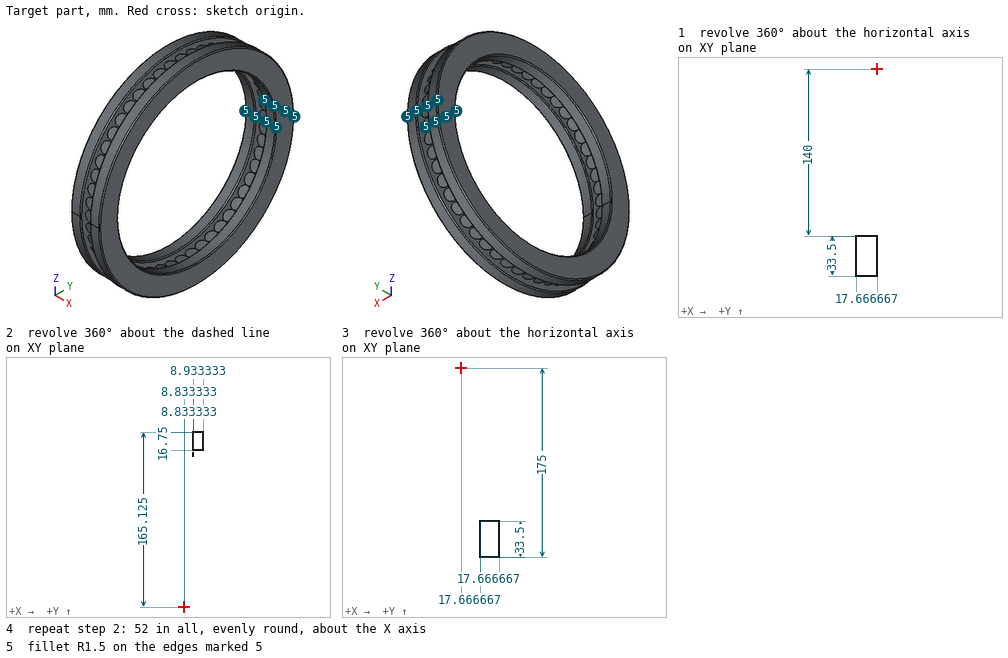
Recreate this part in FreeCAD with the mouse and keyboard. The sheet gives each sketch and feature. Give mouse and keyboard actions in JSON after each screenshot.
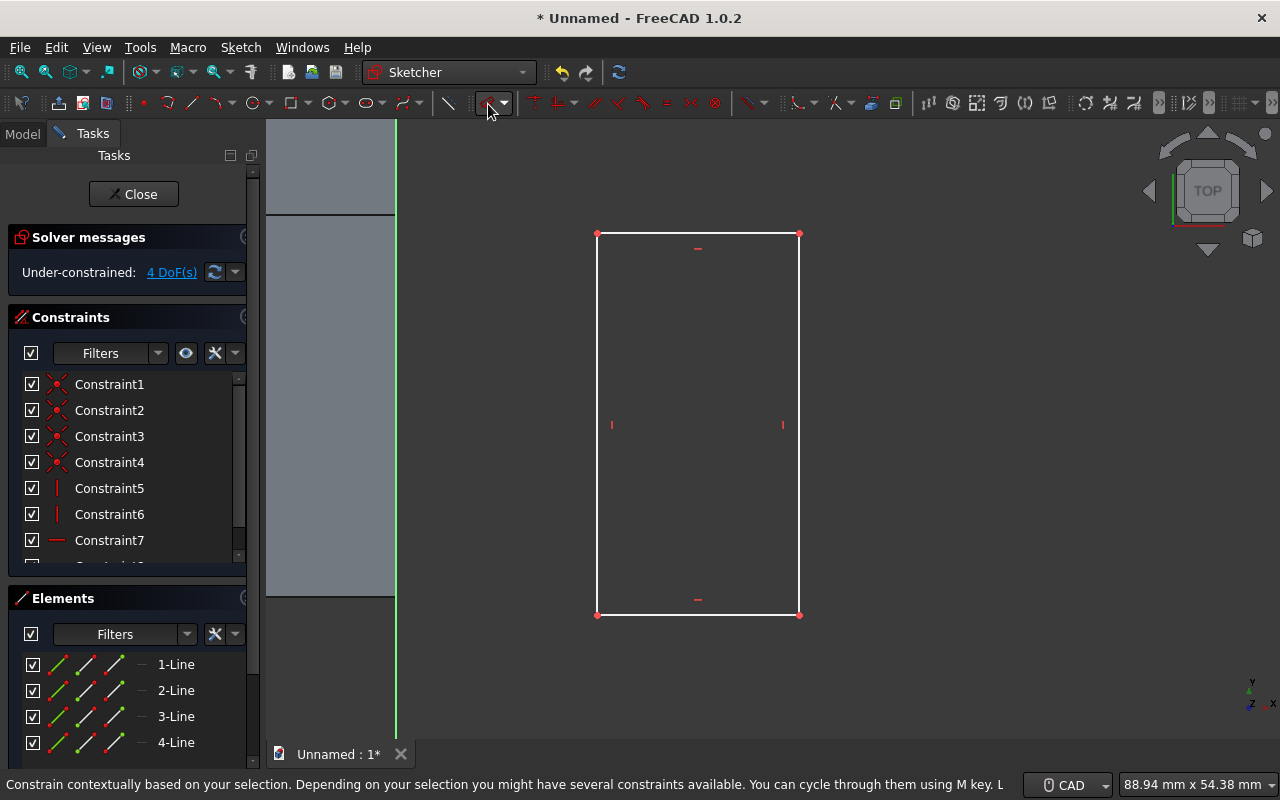
{"action": "left_click", "coordinate": [597, 348]}
{"action": "left_click", "coordinate": [563, 424]}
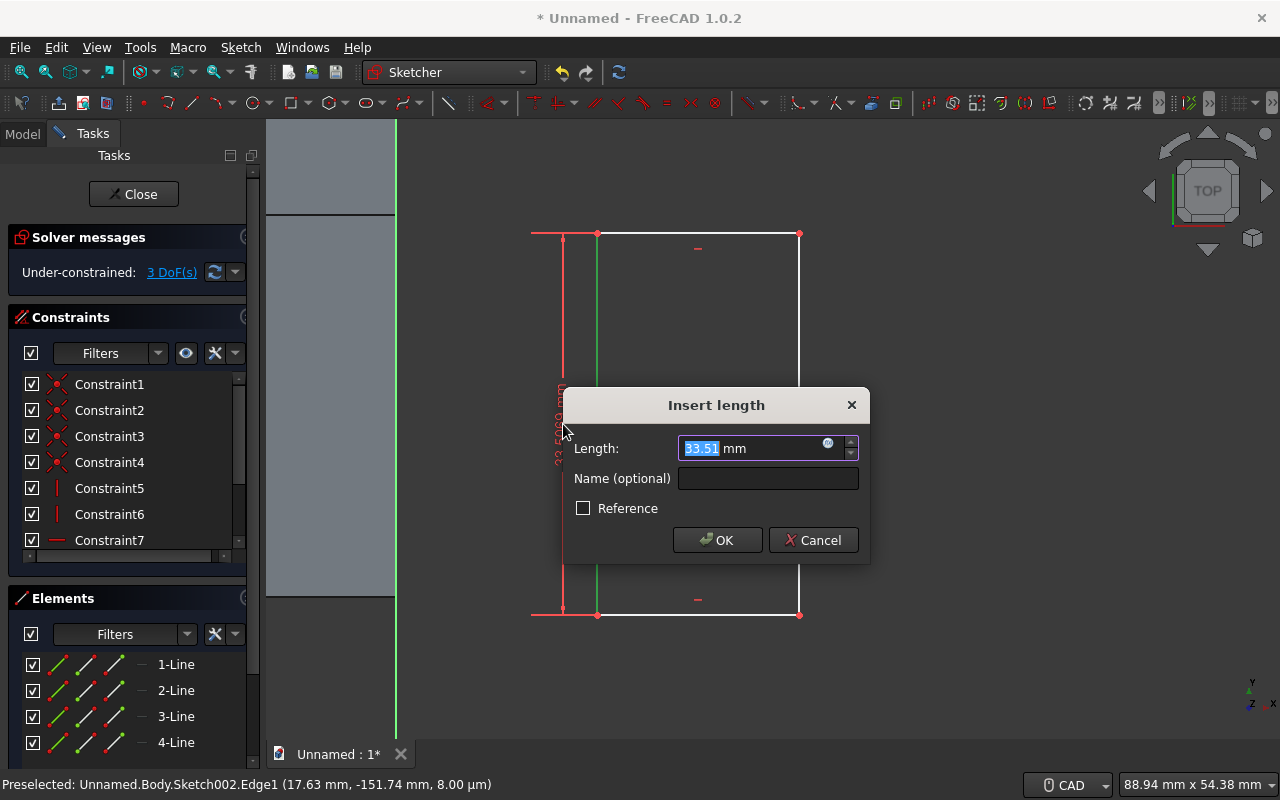
{"action": "type", "text": "33.5"}
{"action": "key", "text": "Return"}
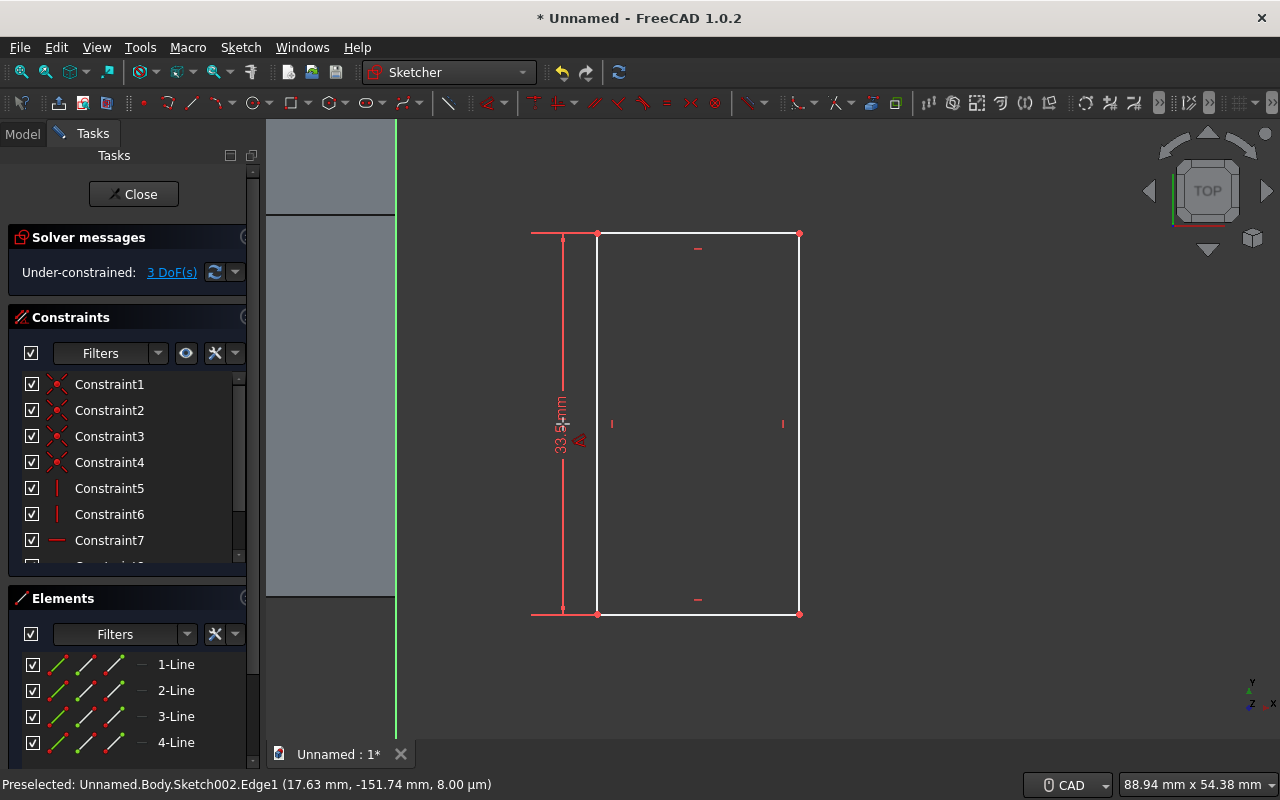
{"action": "left_click", "coordinate": [597, 615]}
{"action": "left_click", "coordinate": [362, 381]}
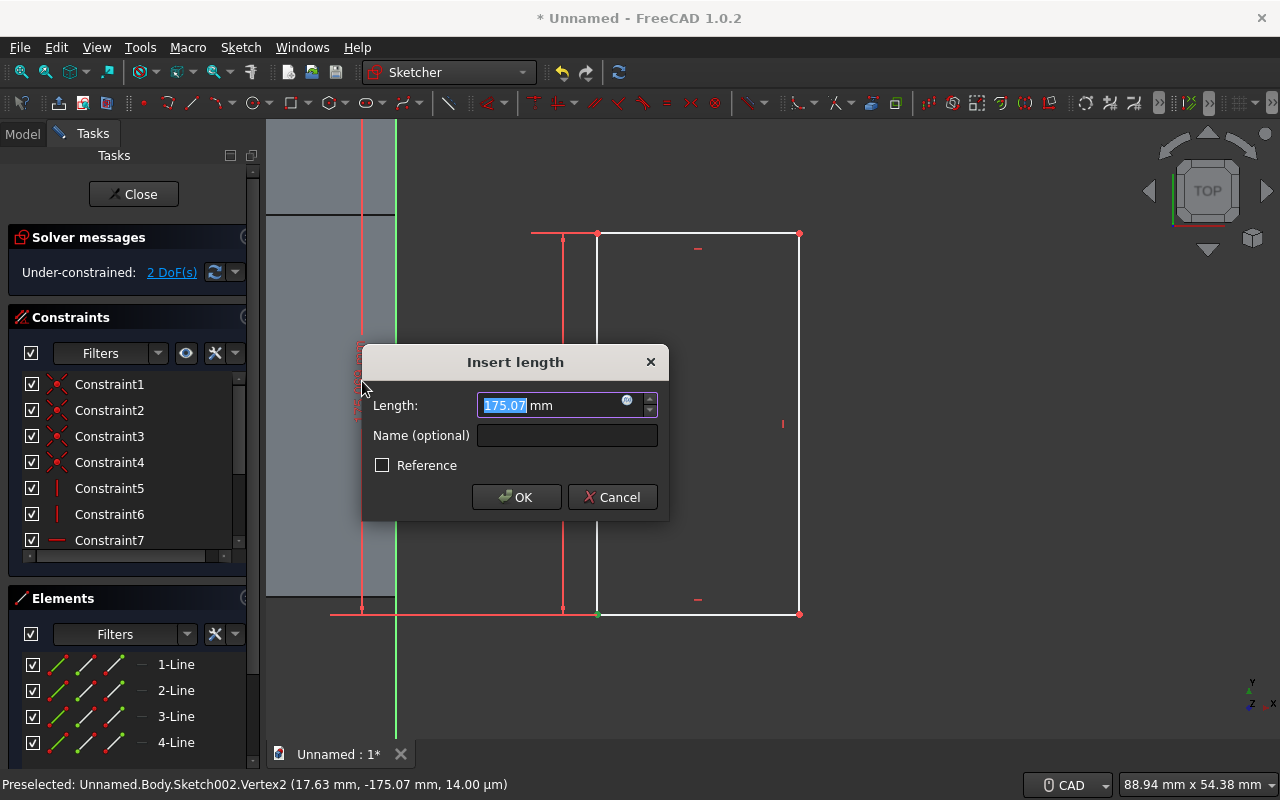
{"action": "type", "text": "175"}
{"action": "key", "text": "Return"}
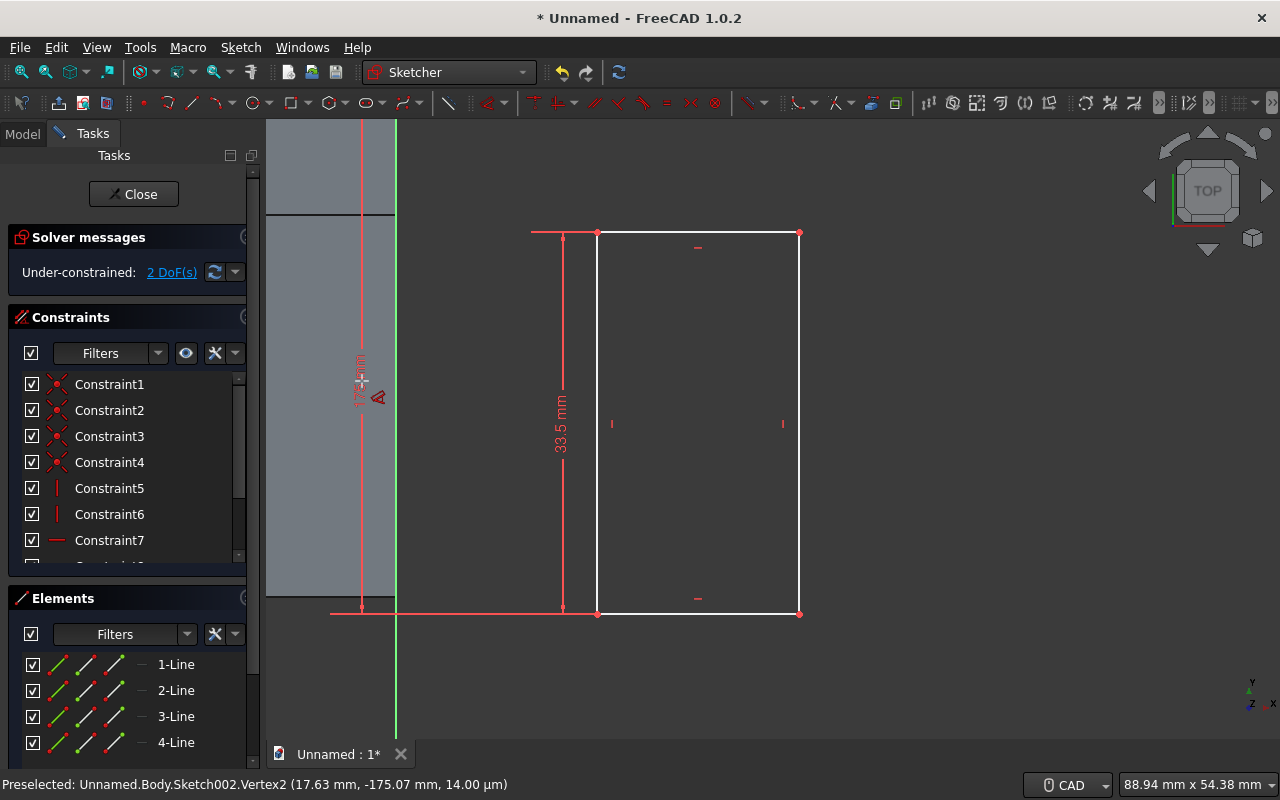
{"action": "left_click", "coordinate": [658, 614]}
{"action": "left_click", "coordinate": [698, 648]}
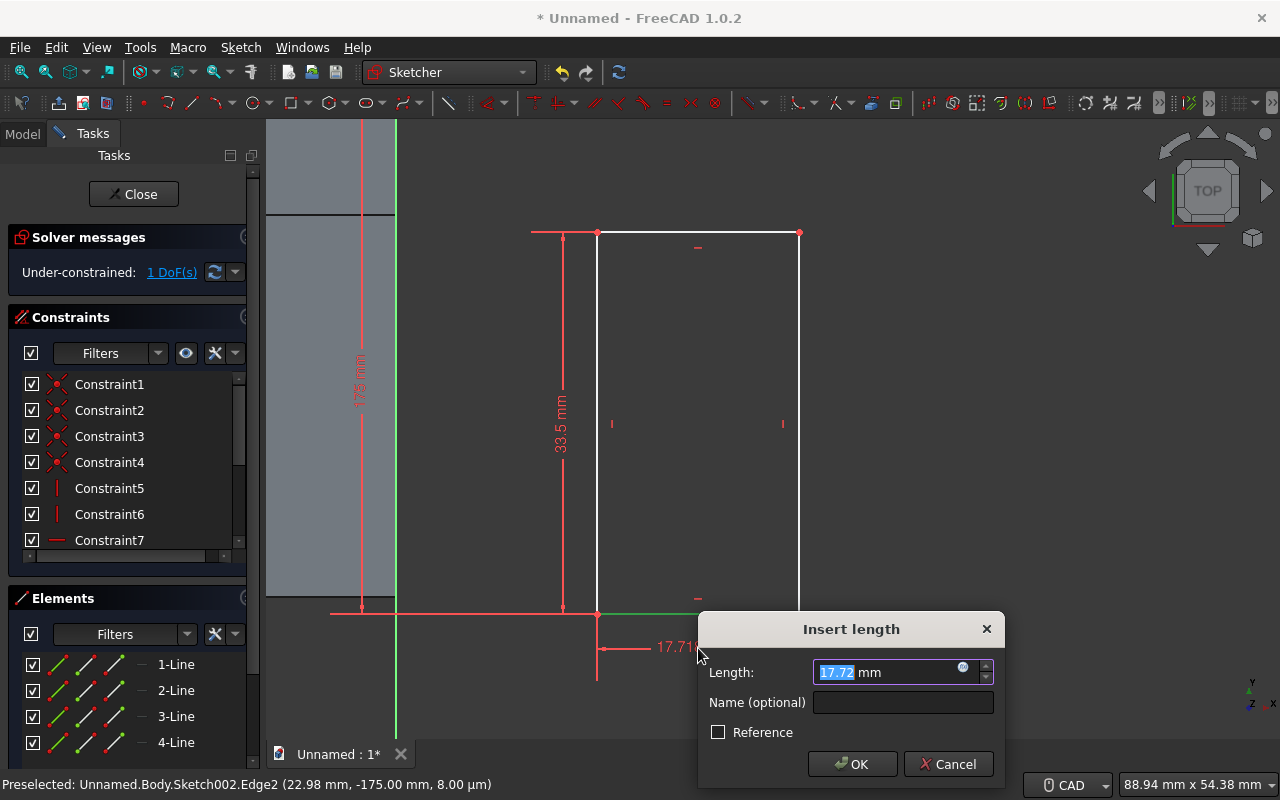
{"action": "type", "text": "17.666667"}
{"action": "key", "text": "Return"}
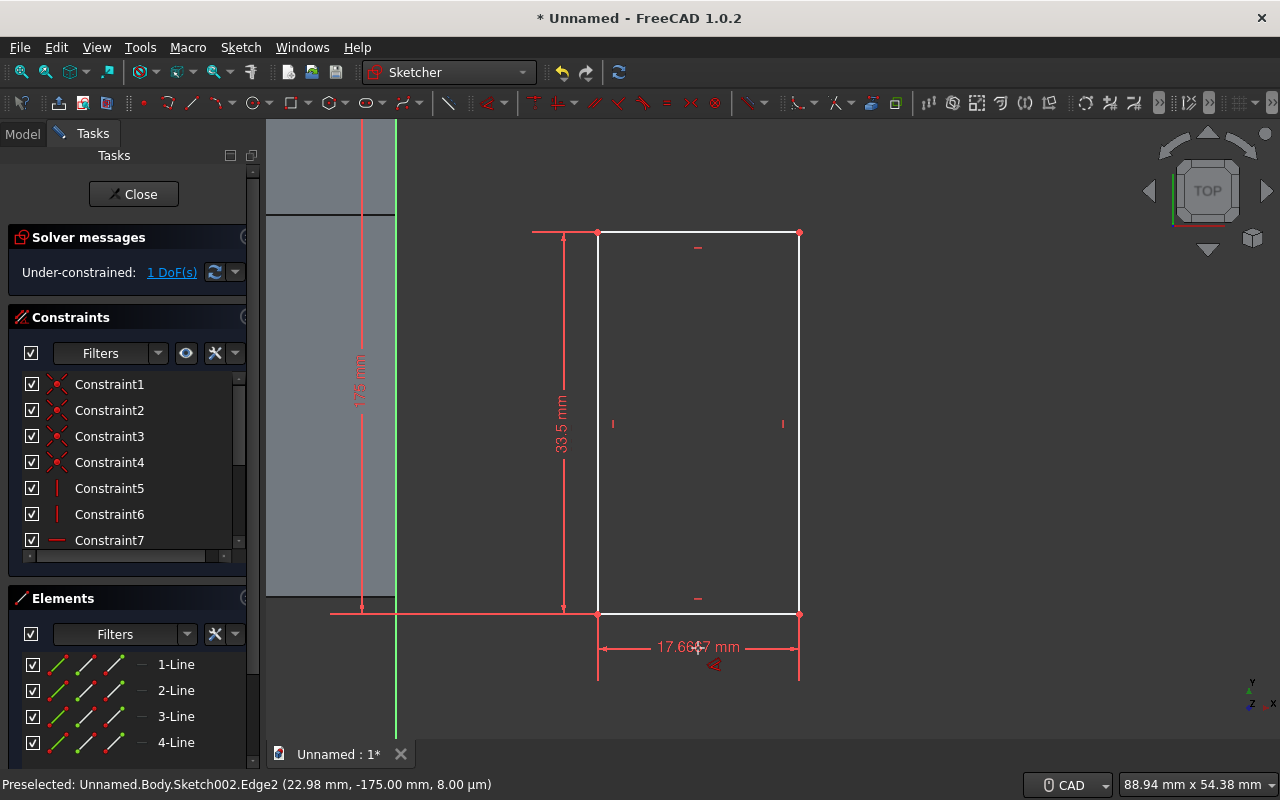
{"action": "left_click", "coordinate": [598, 232]}
{"action": "left_click", "coordinate": [497, 266]}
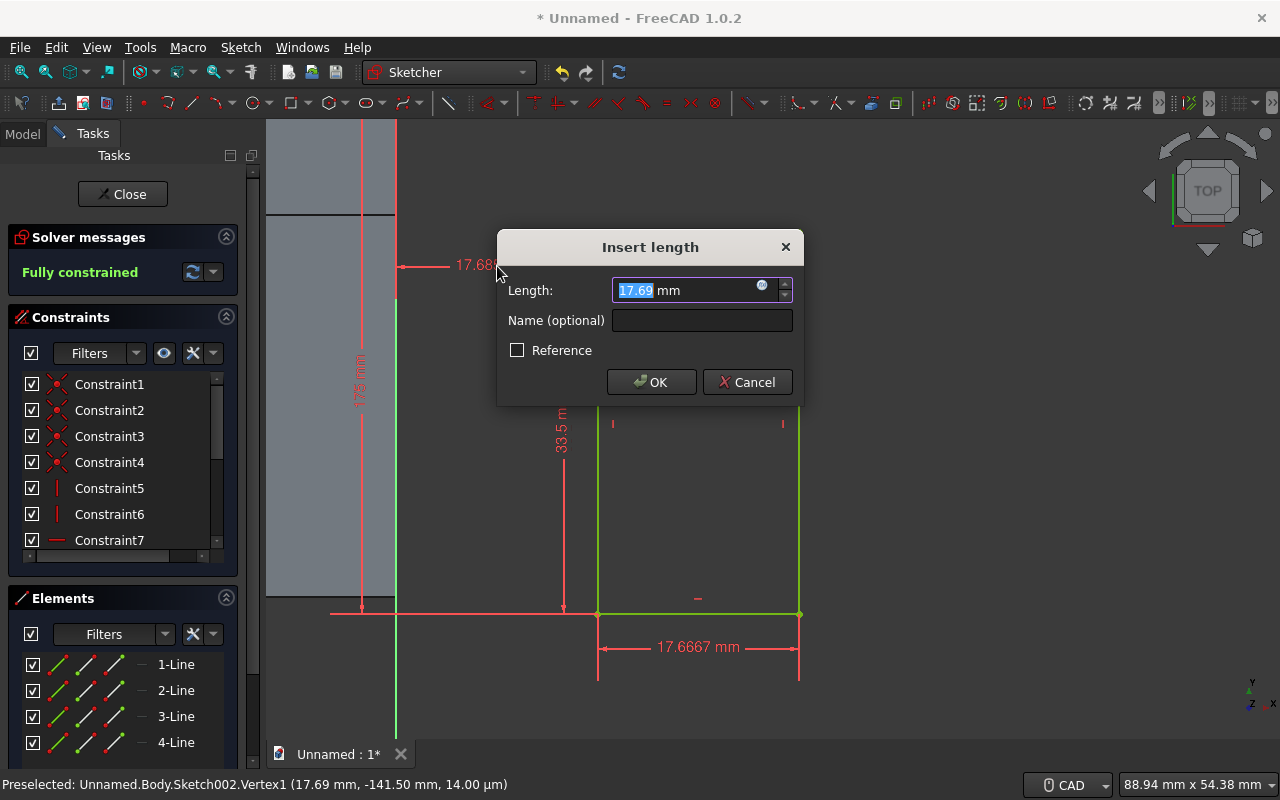
{"action": "type", "text": "17.666667"}
{"action": "key", "text": "Return"}
{"action": "key", "text": "Escape"}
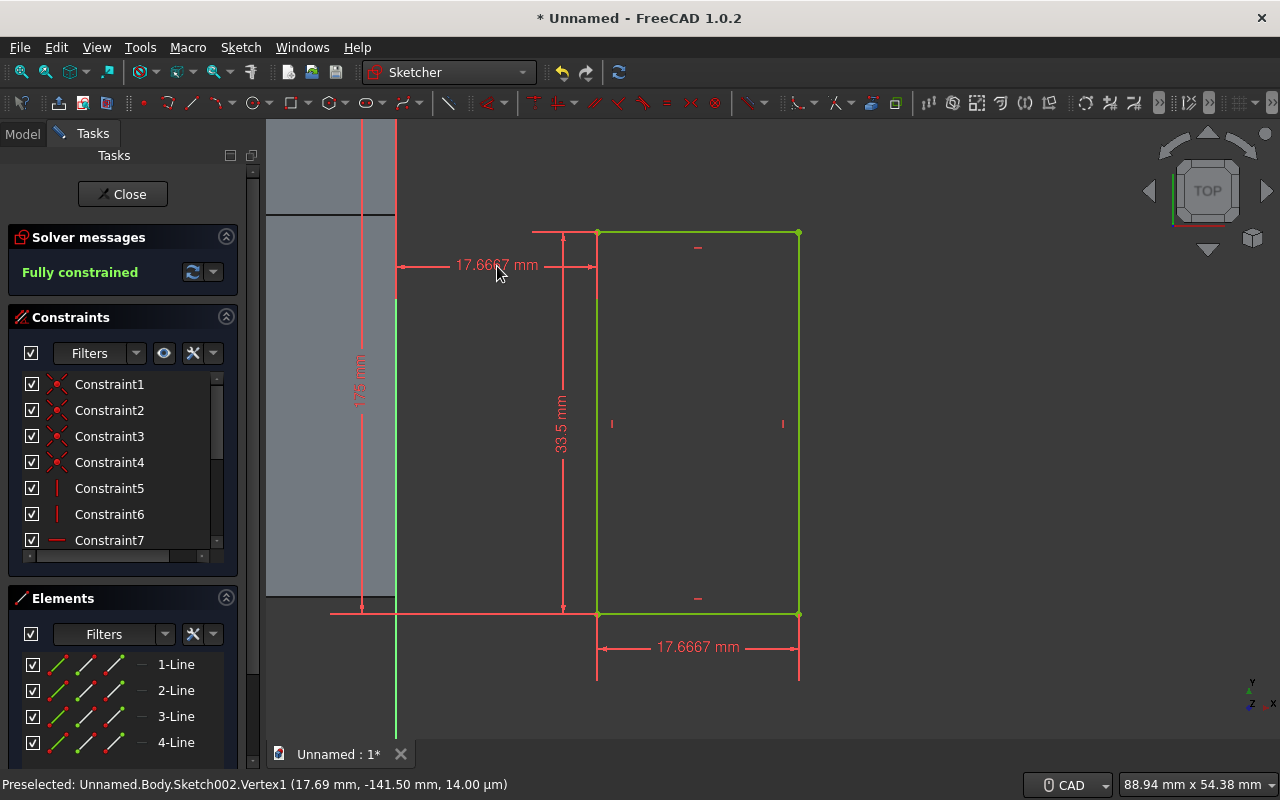
{"action": "left_click", "coordinate": [123, 194]}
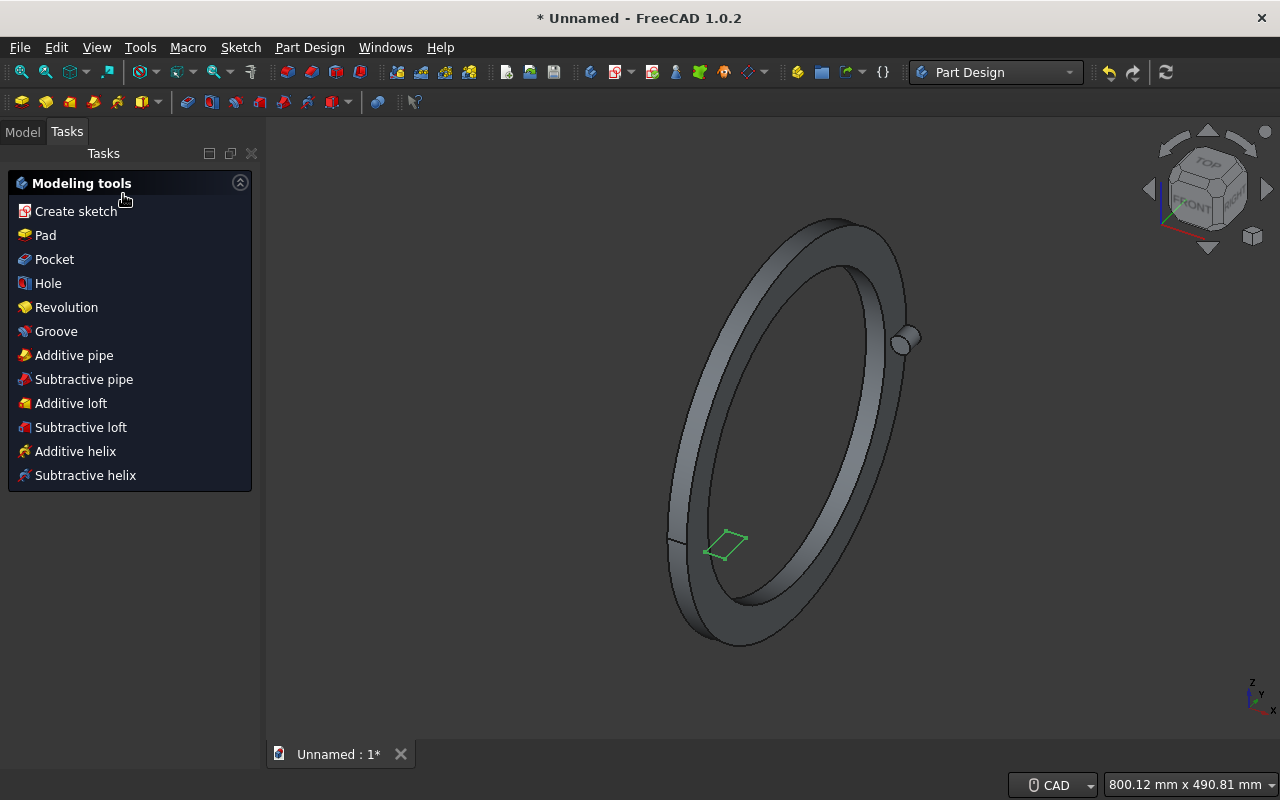
{"action": "left_click", "coordinate": [46, 102]}